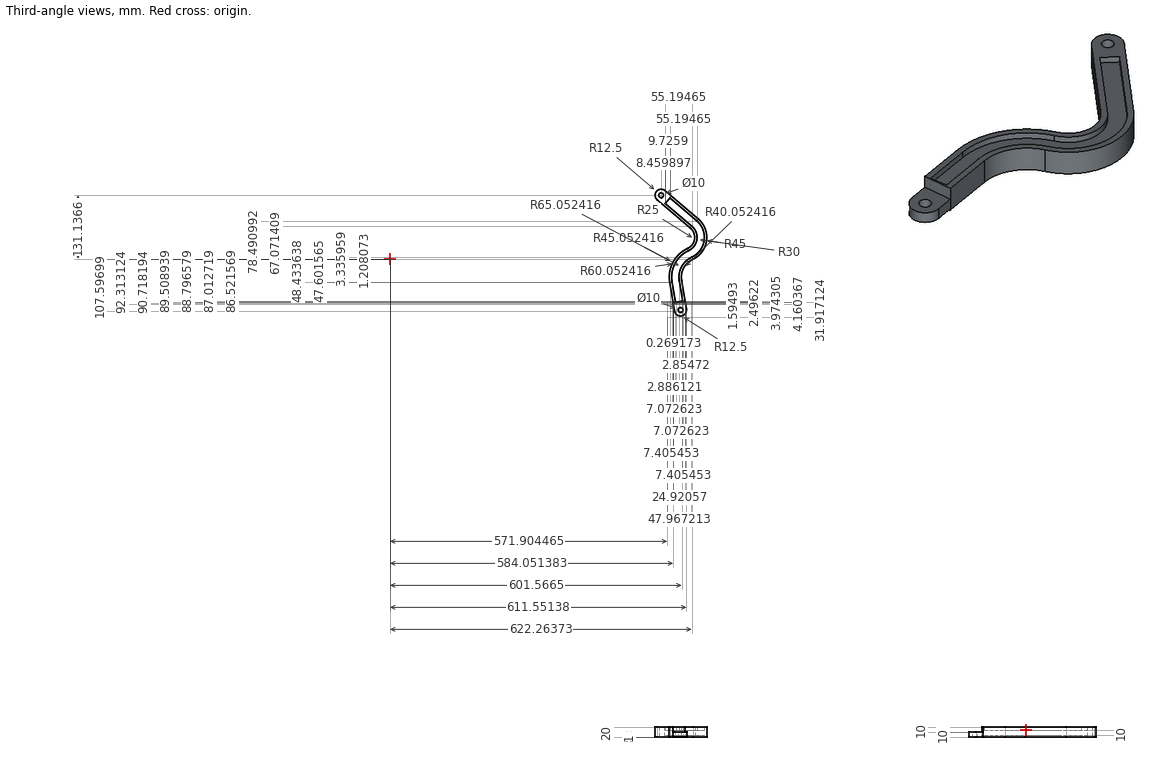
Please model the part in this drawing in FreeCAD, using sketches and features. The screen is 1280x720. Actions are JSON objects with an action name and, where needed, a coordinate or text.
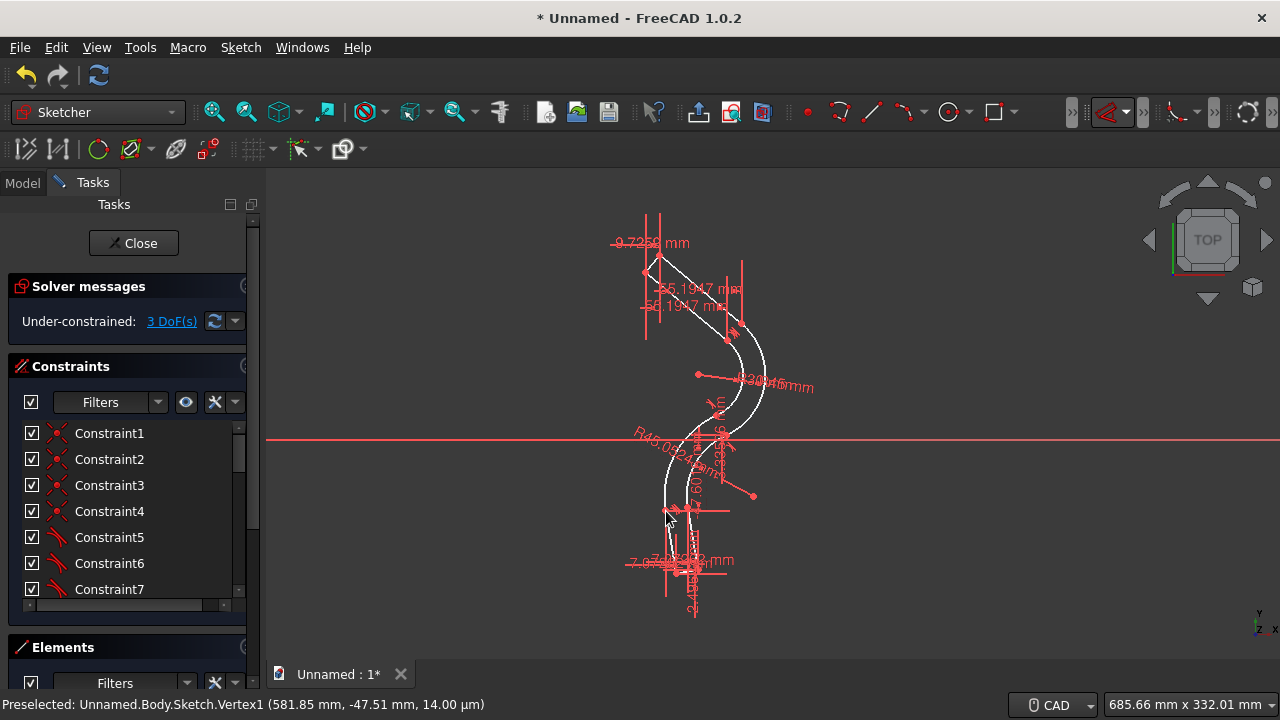
{"action": "left_click", "coordinate": [676, 574]}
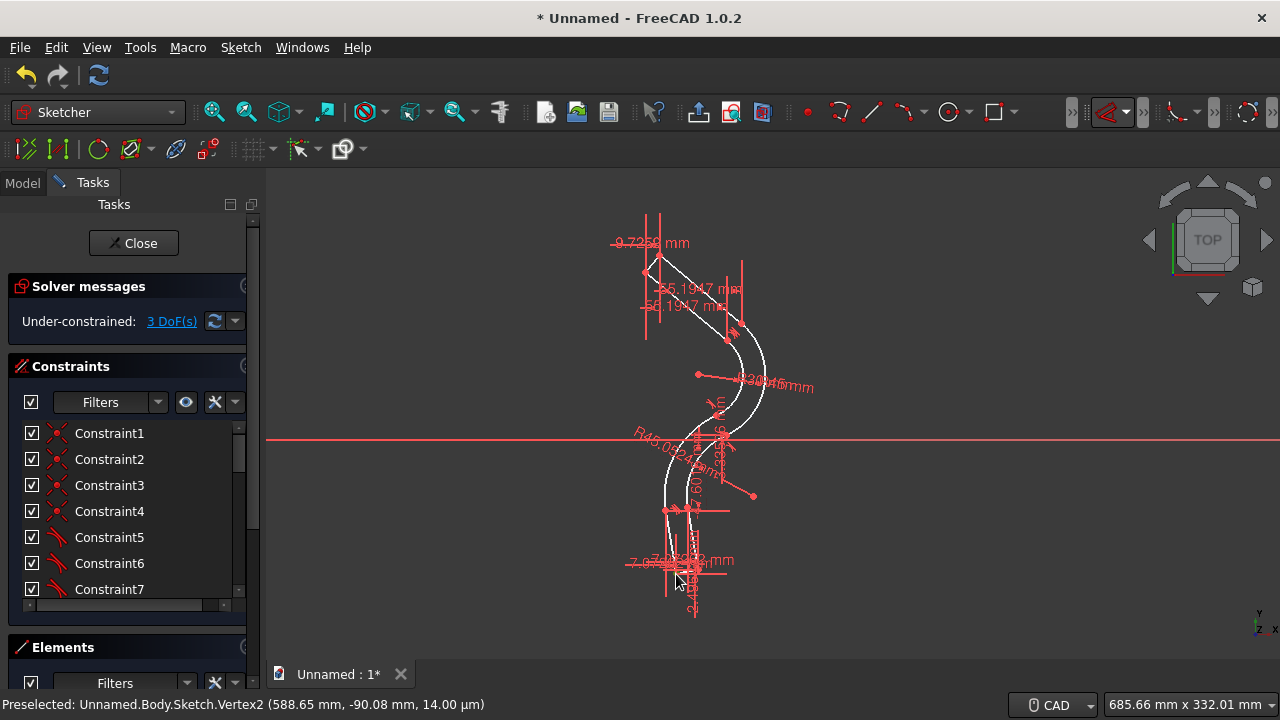
{"action": "left_click", "coordinate": [1128, 112]}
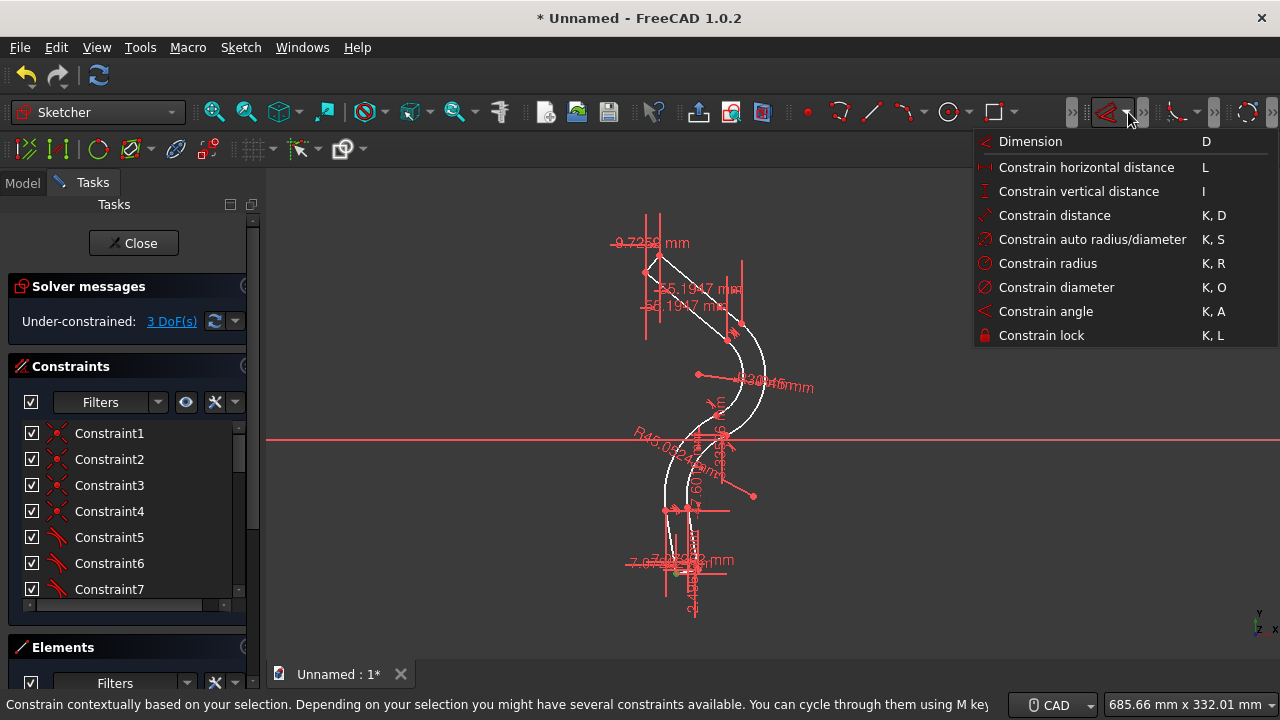
{"action": "left_click", "coordinate": [1126, 191]}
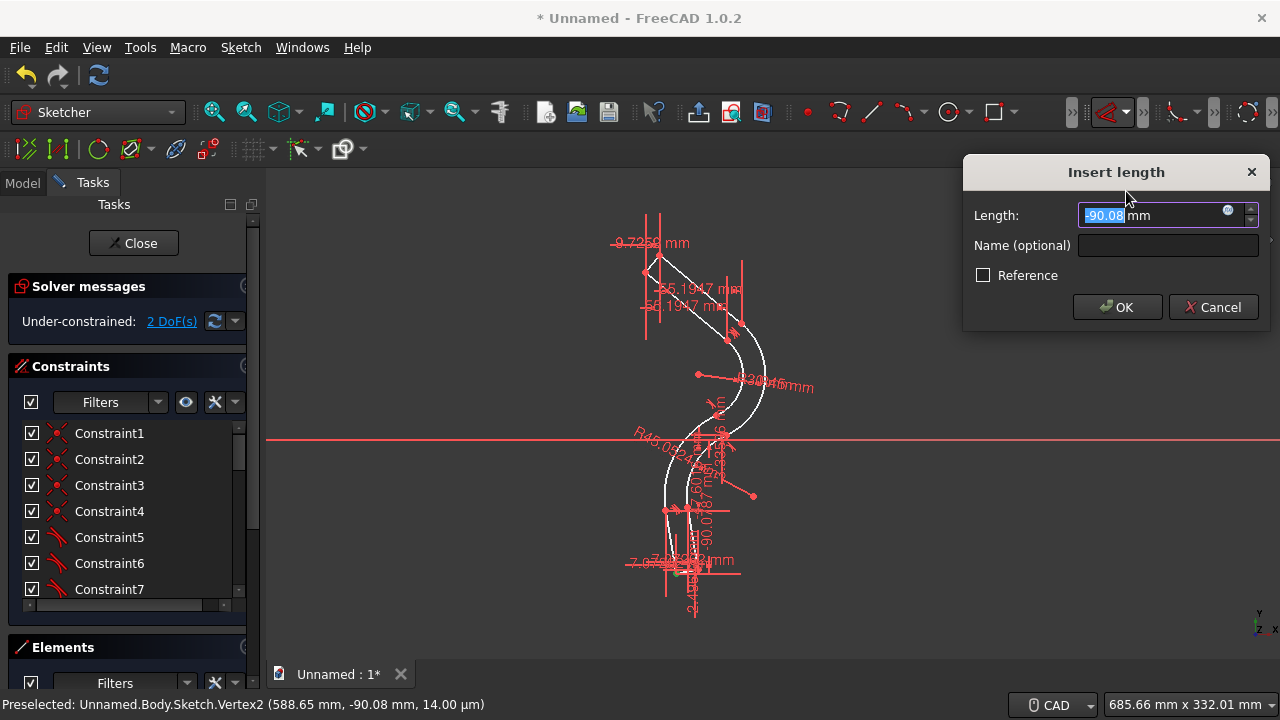
{"action": "type", "text": "-89.508939"}
{"action": "key", "text": "Return"}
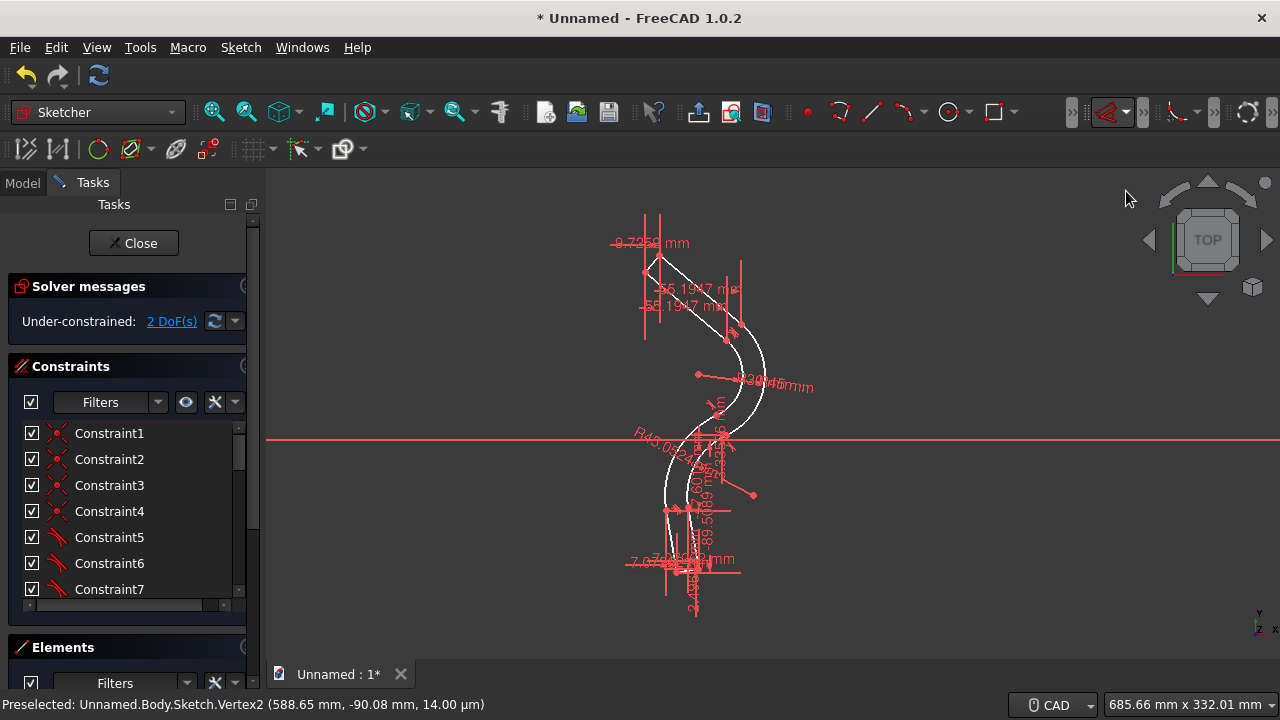
{"action": "left_click", "coordinate": [741, 324]}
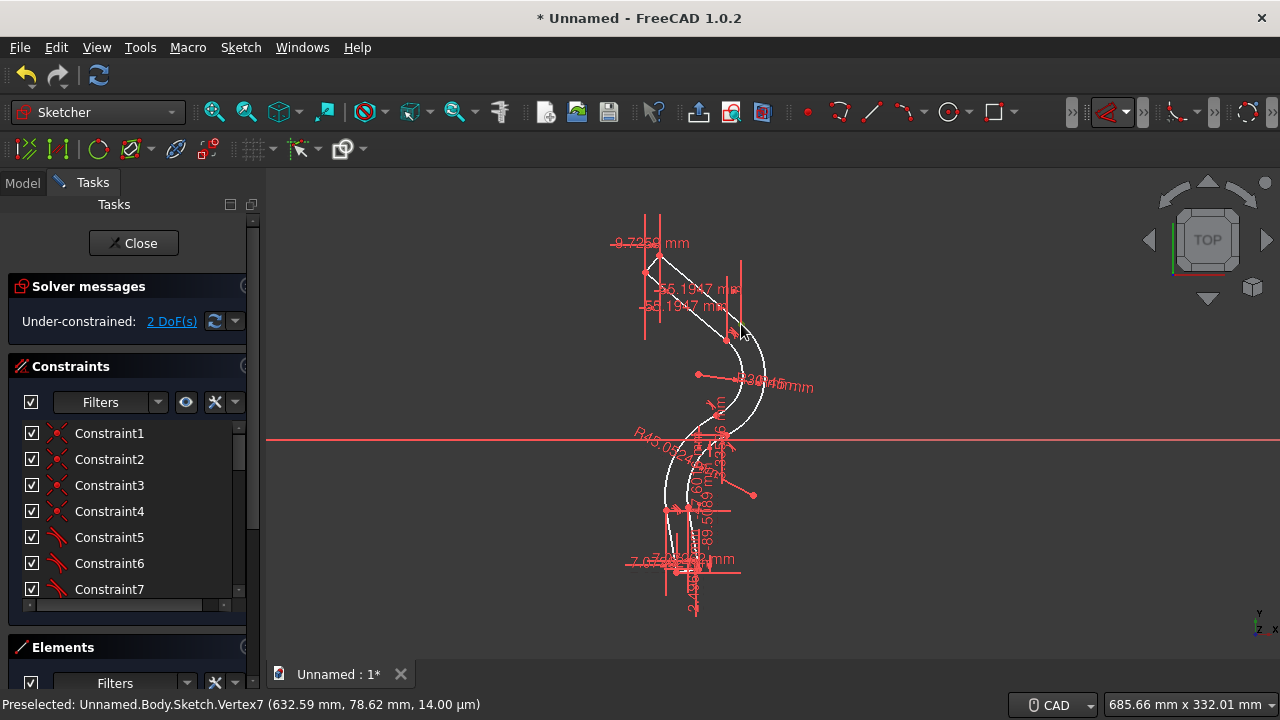
{"action": "left_click", "coordinate": [1128, 112]}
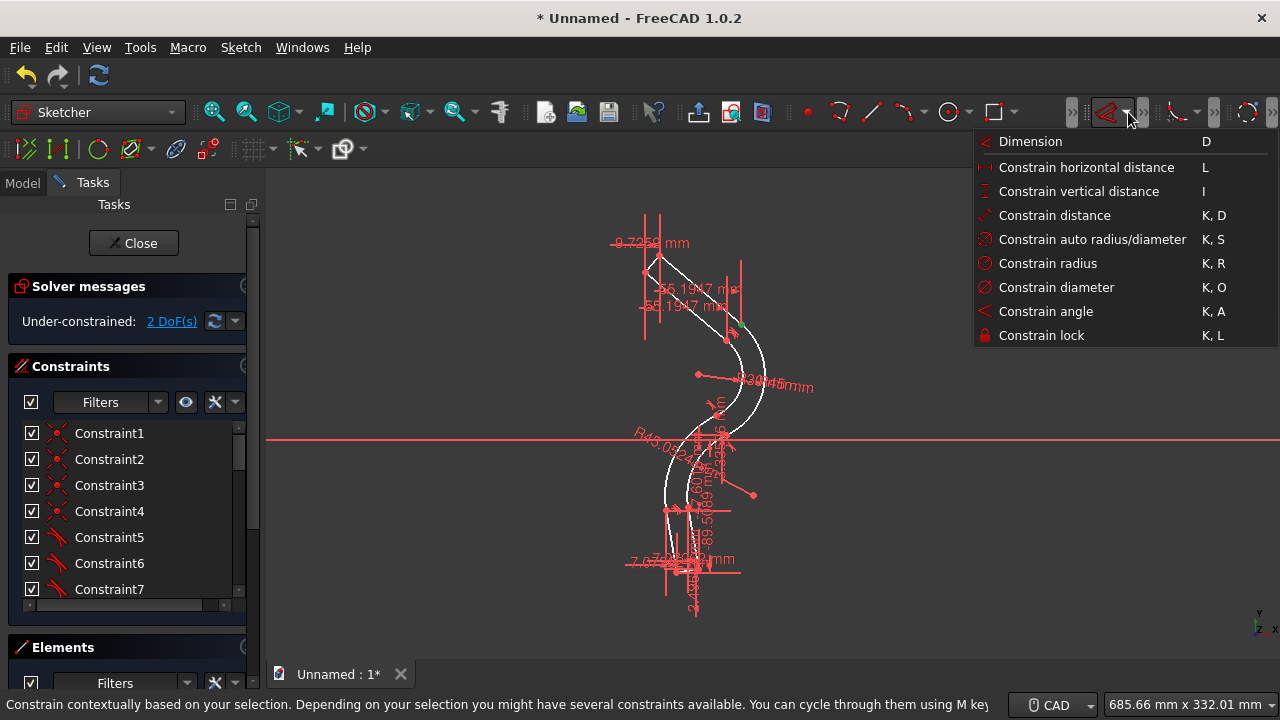
{"action": "left_click", "coordinate": [1126, 191]}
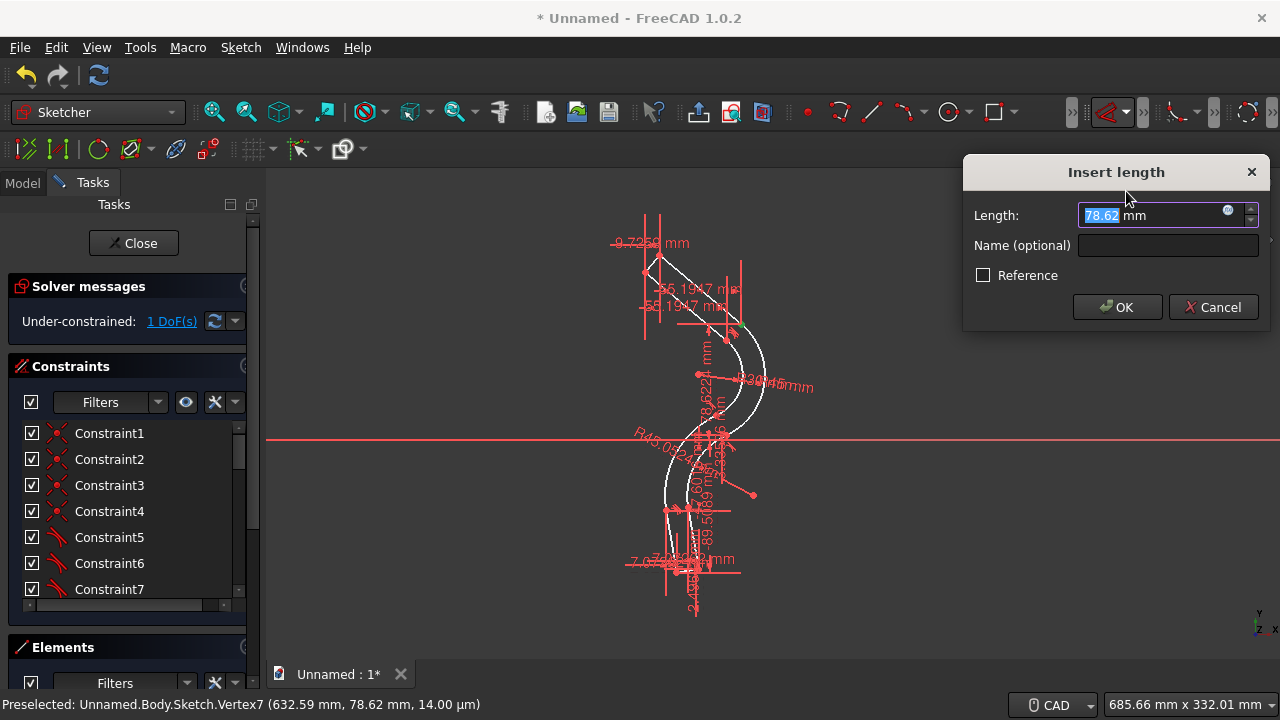
{"action": "type", "text": "78.490992"}
{"action": "key", "text": "Return"}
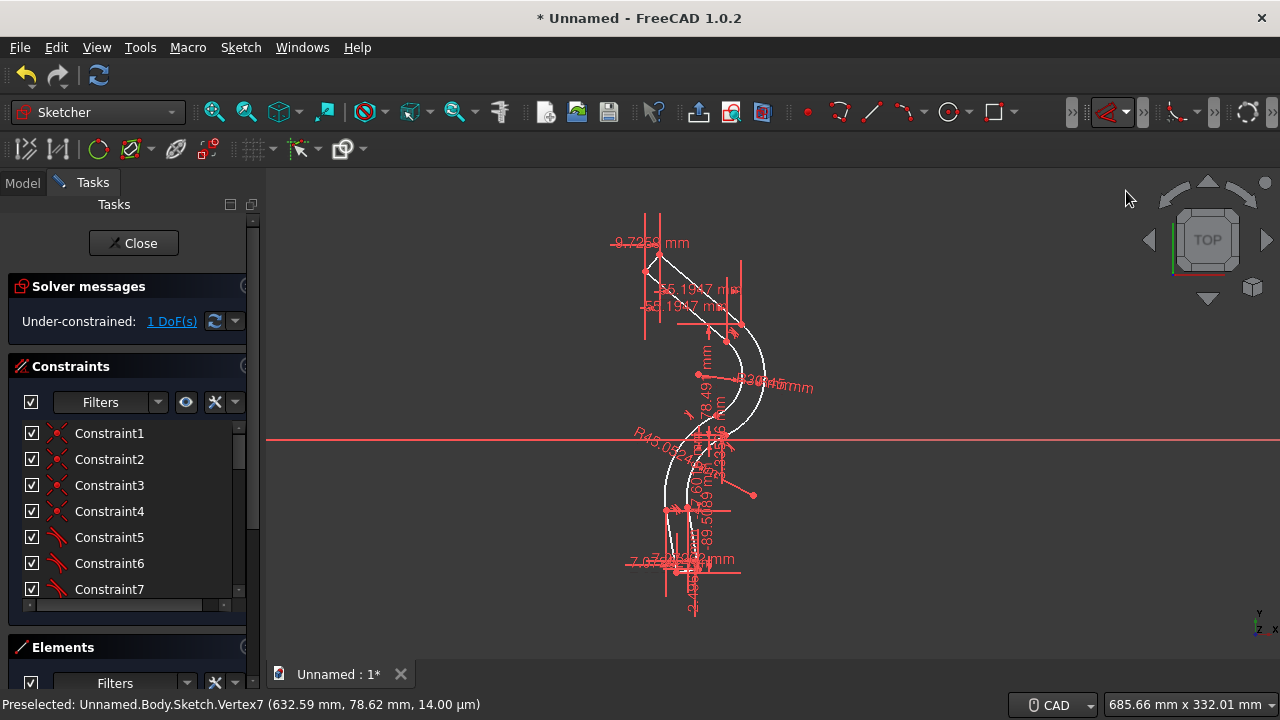
{"action": "left_click", "coordinate": [726, 435]}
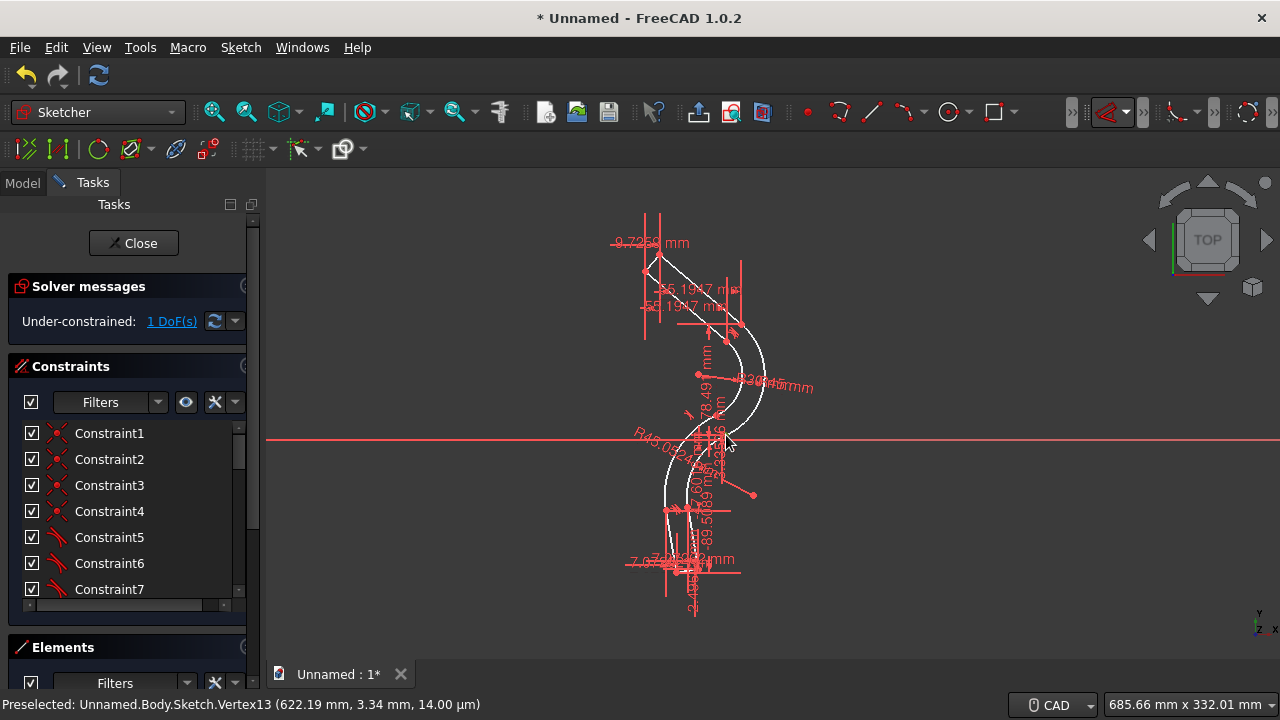
{"action": "key", "text": "l"}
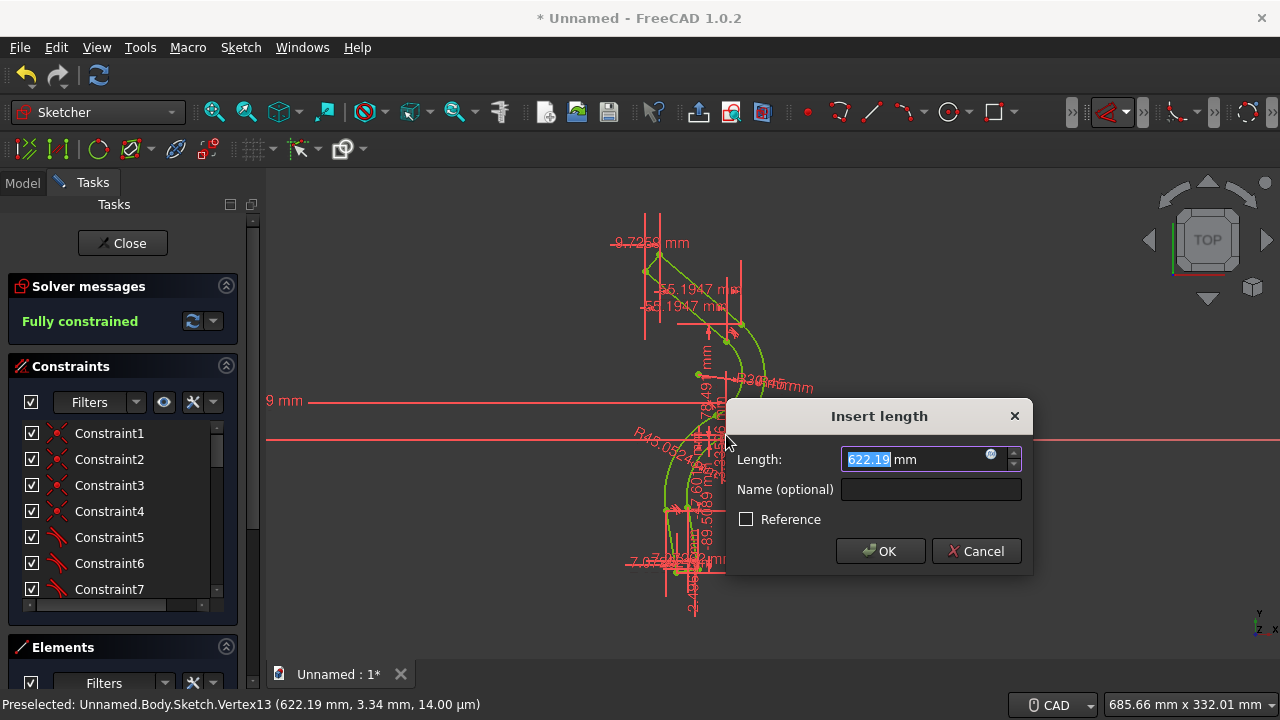
{"action": "type", "text": "622.26373"}
{"action": "key", "text": "Return"}